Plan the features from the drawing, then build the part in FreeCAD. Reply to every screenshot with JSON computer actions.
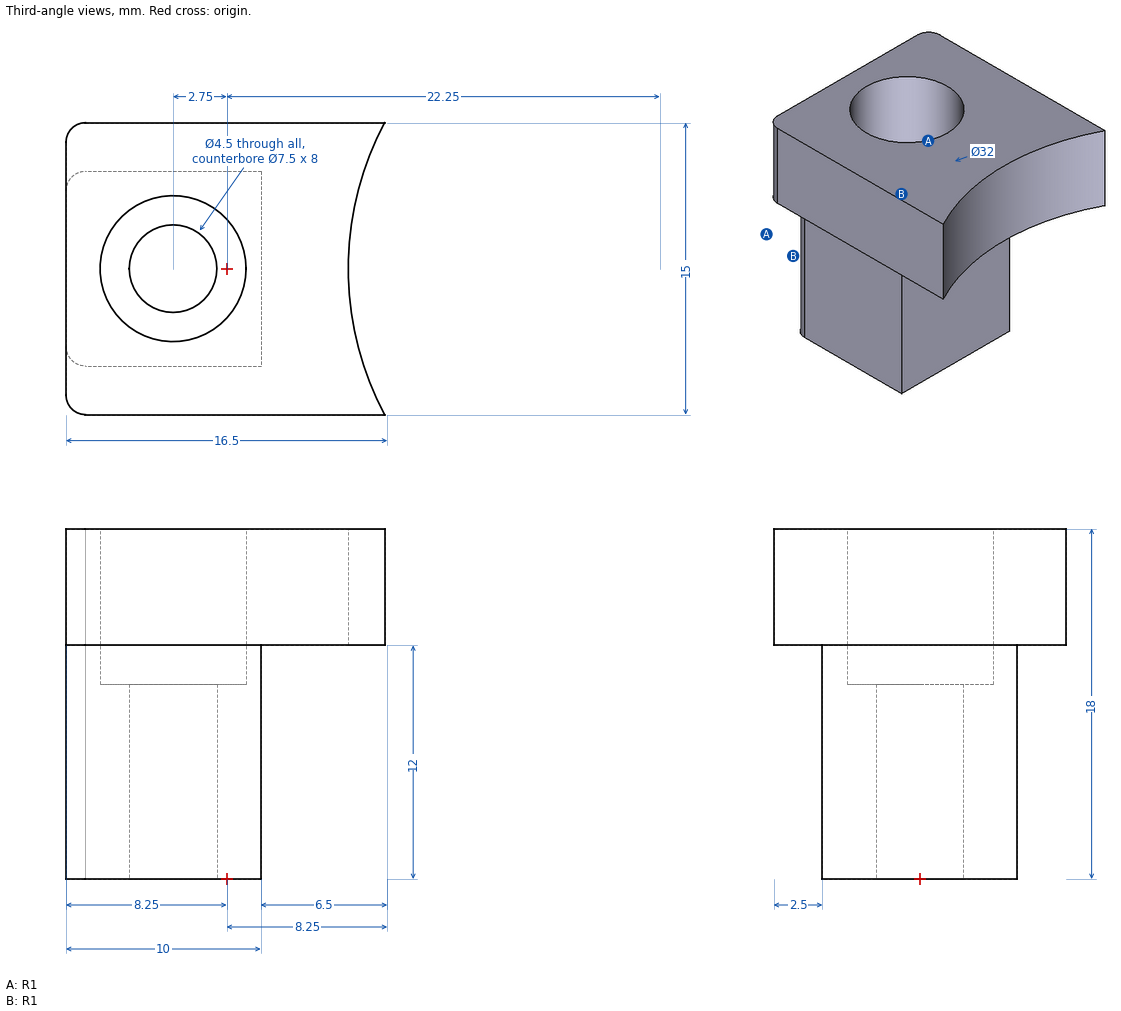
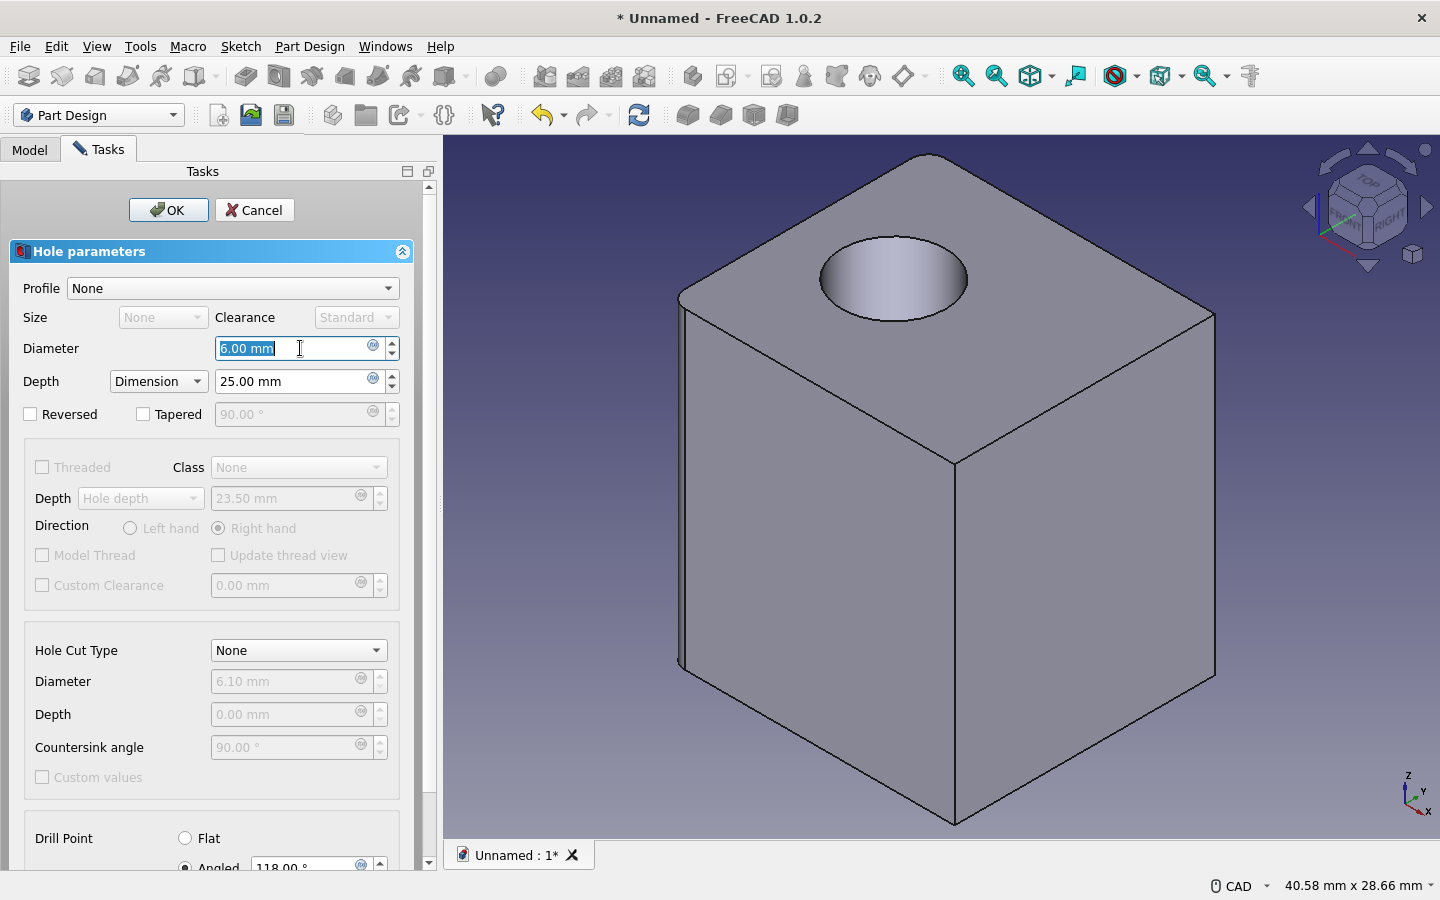
{"action": "type", "text": "4.5"}
{"action": "key", "text": "Tab"}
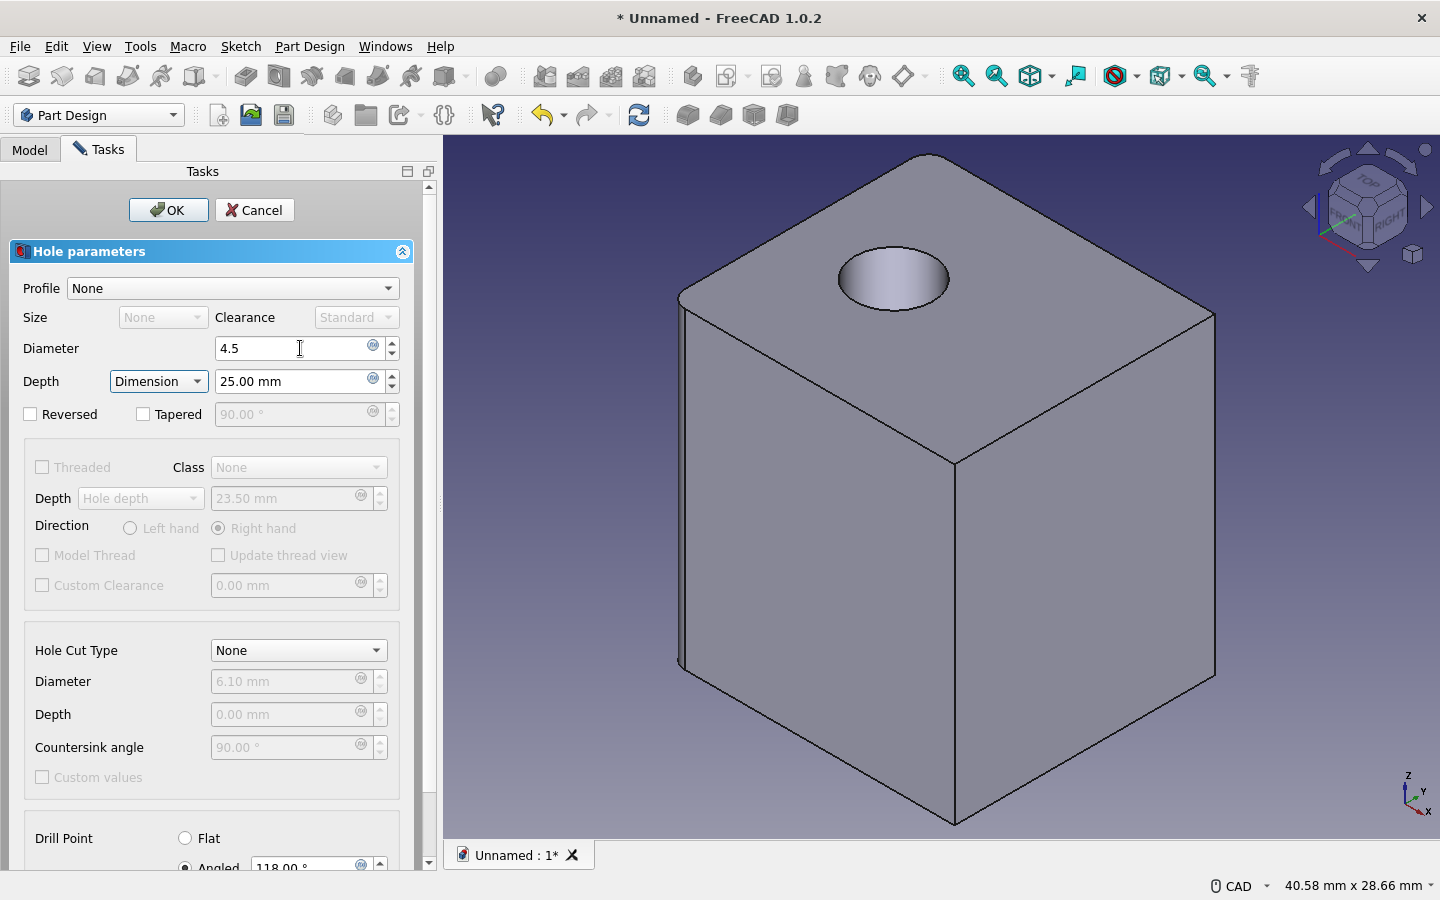
{"action": "left_click", "coordinate": [160, 382]}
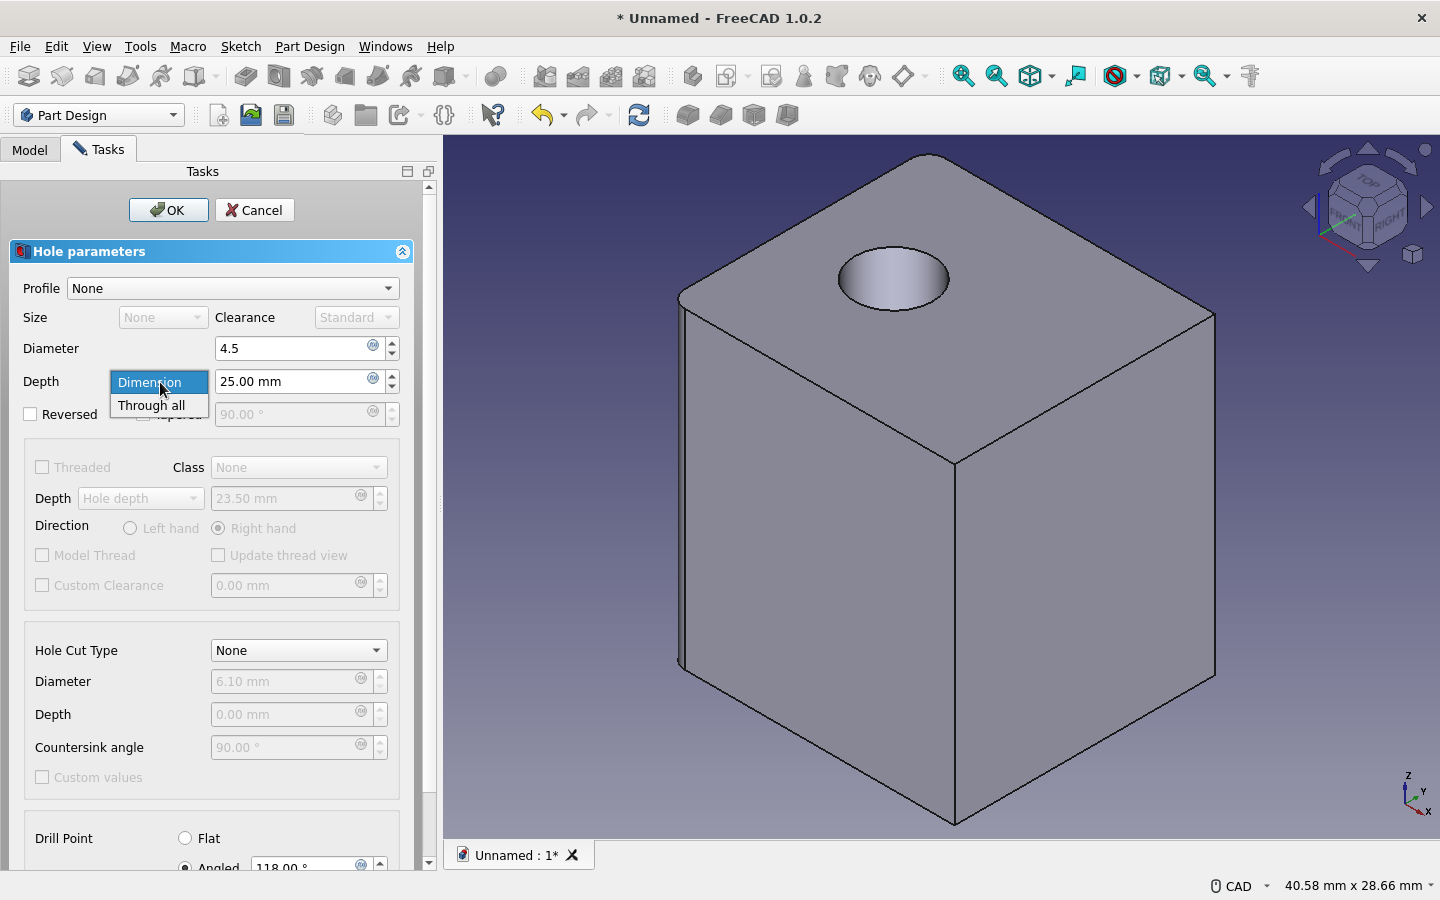
{"action": "left_click", "coordinate": [158, 406]}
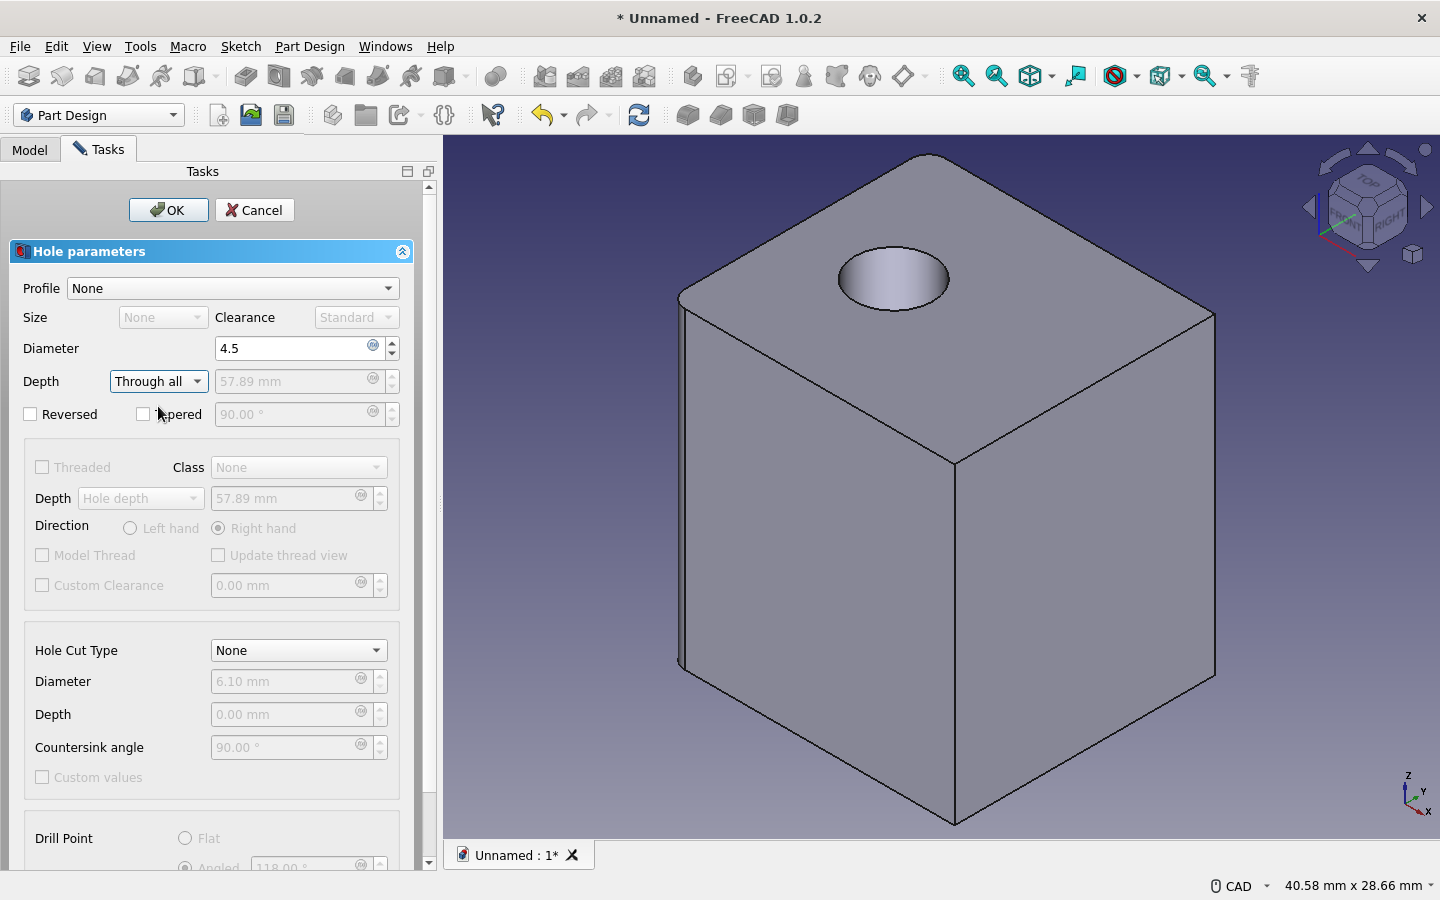
{"action": "left_click", "coordinate": [300, 650]}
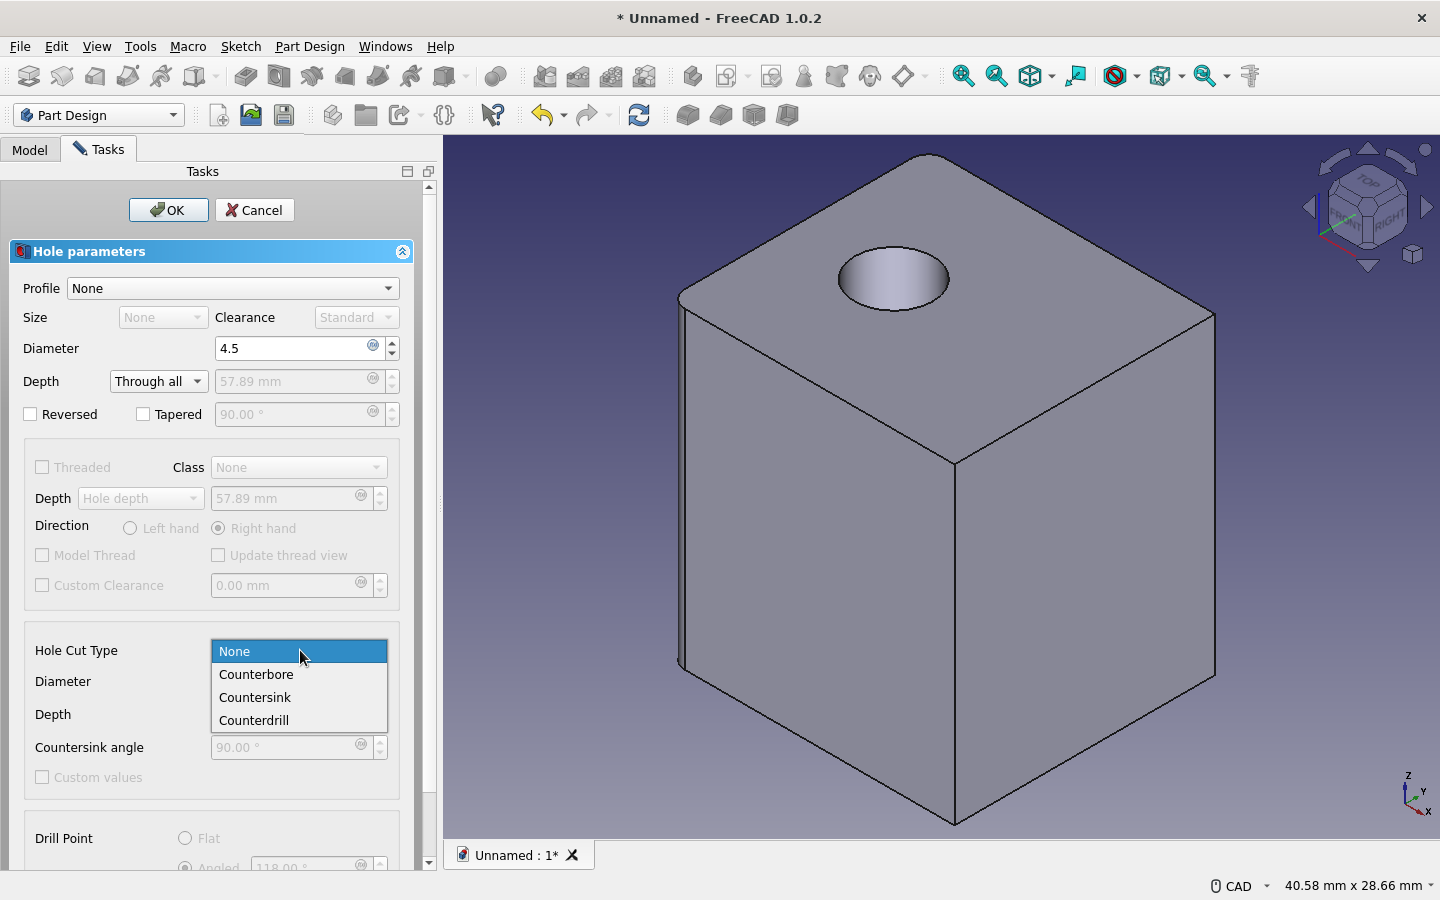
{"action": "left_click", "coordinate": [298, 674]}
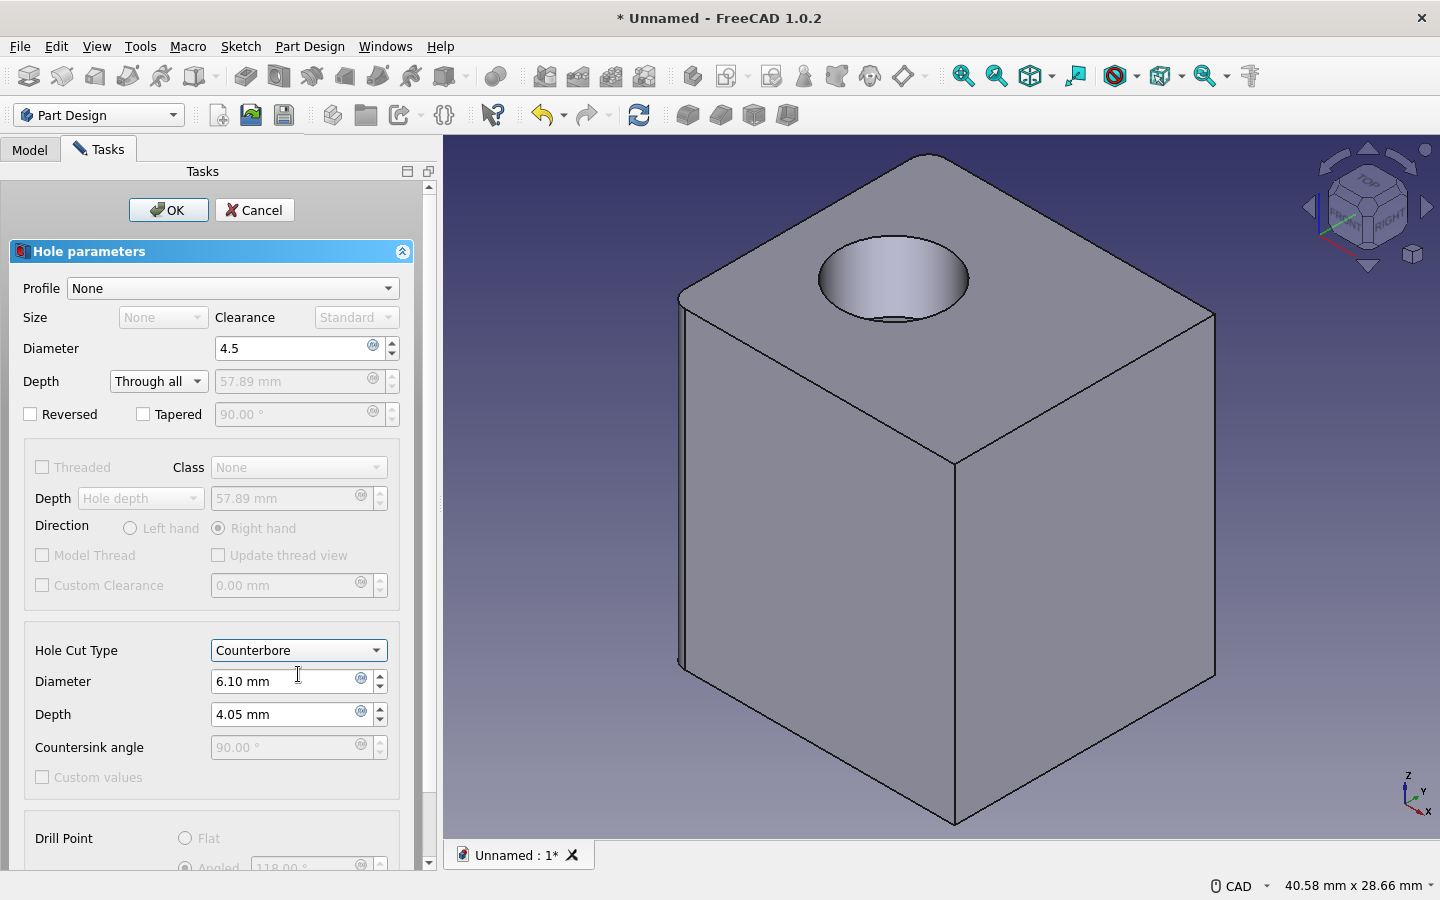
{"action": "triple_click", "coordinate": [292, 682]}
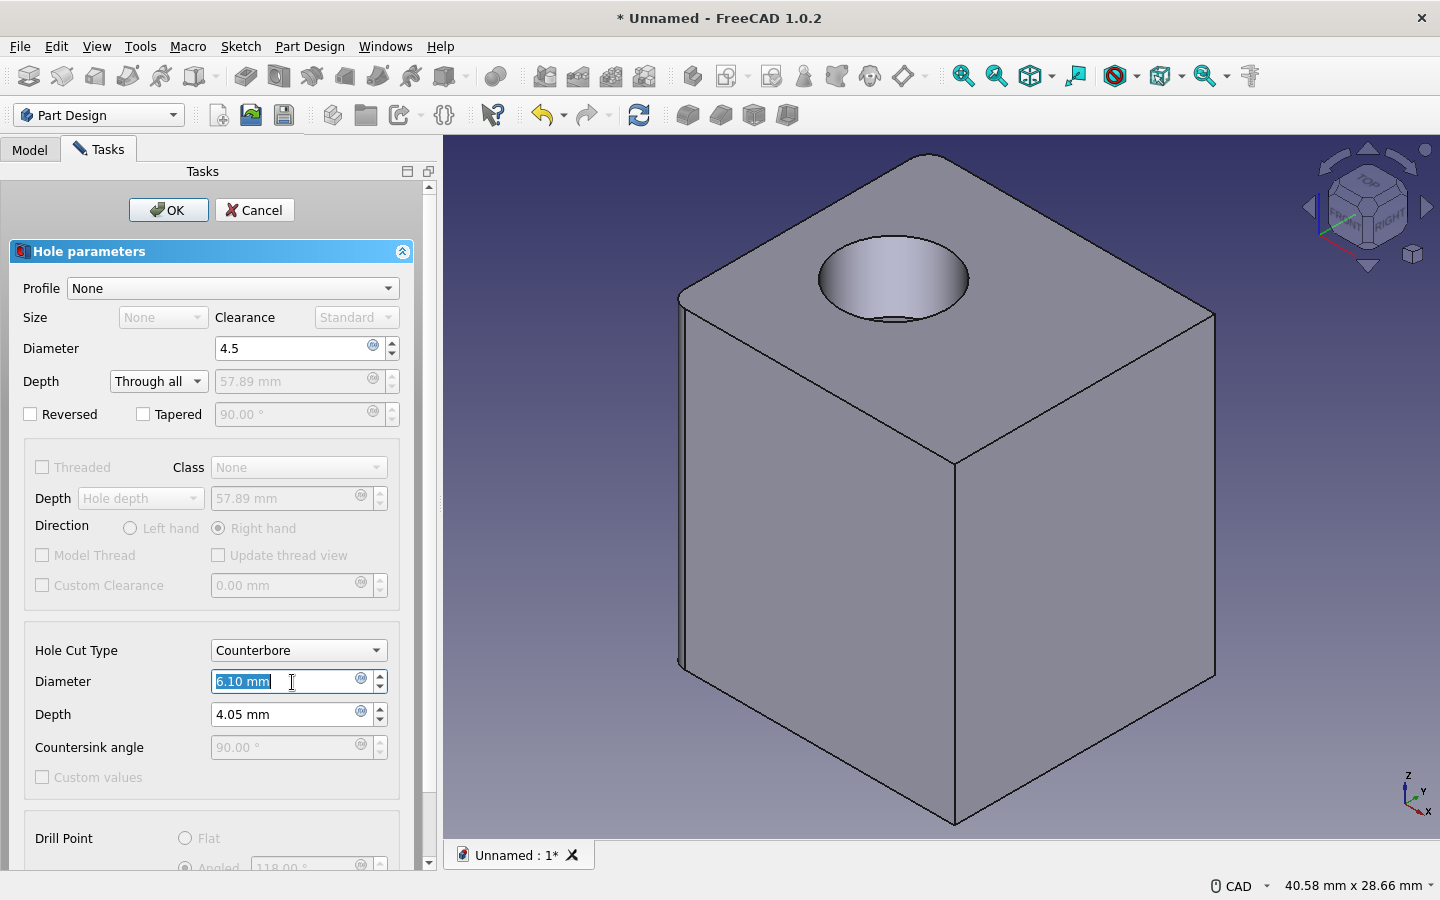
{"action": "type", "text": "7.5"}
{"action": "key", "text": "Tab"}